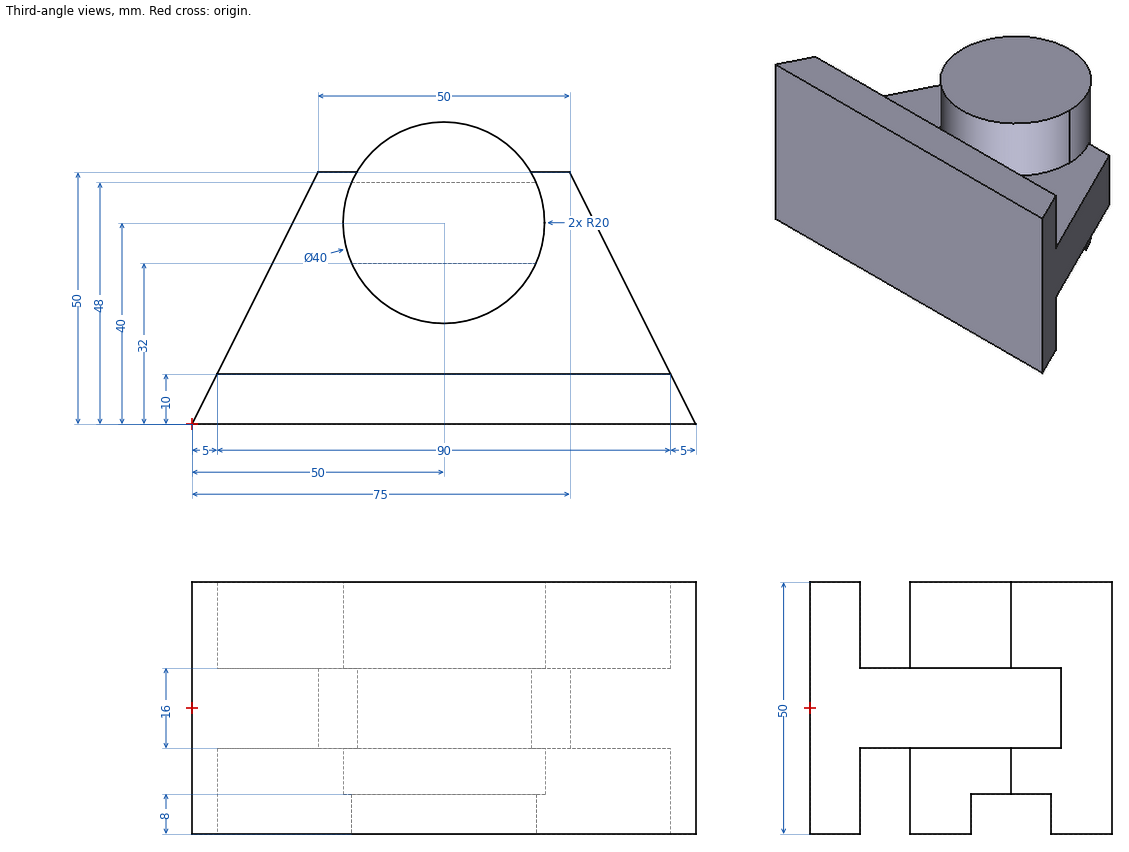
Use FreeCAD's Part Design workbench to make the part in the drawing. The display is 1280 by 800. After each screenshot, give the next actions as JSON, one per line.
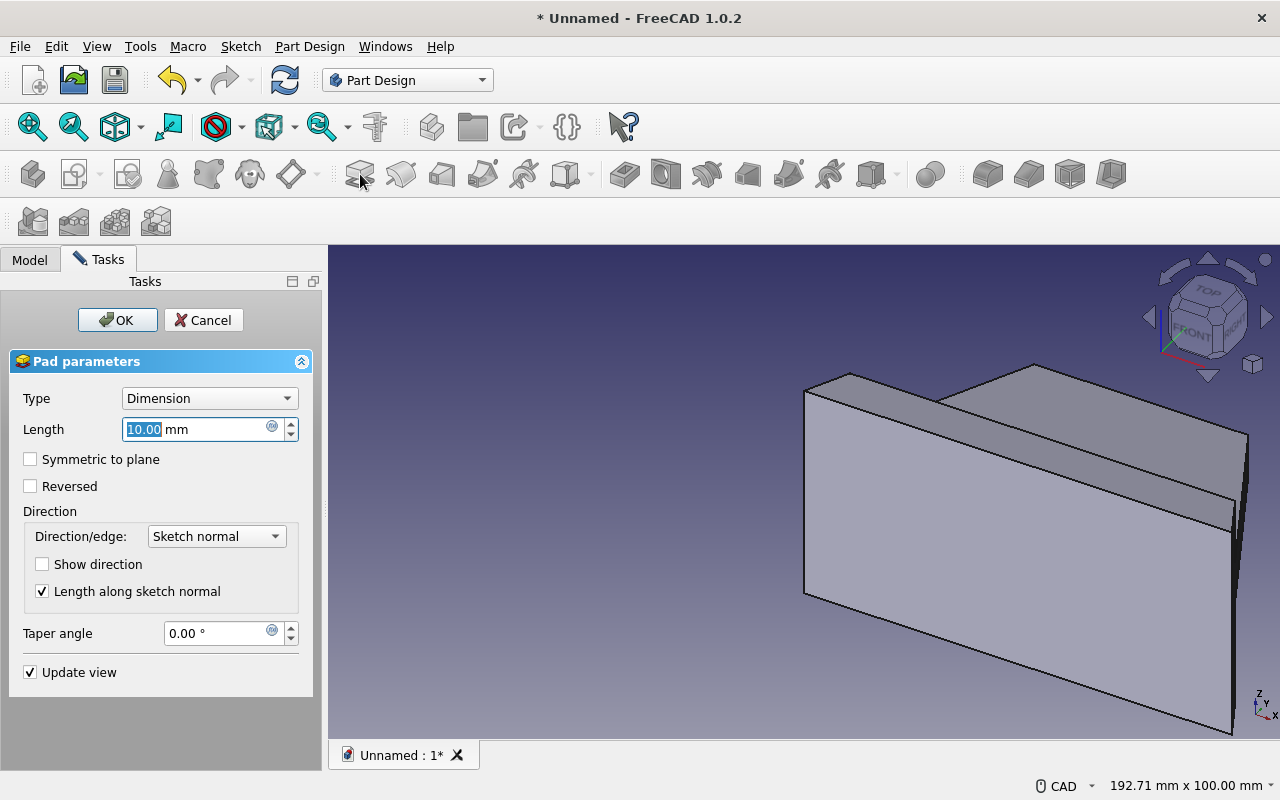
{"action": "type", "text": "16"}
{"action": "key", "text": "Tab"}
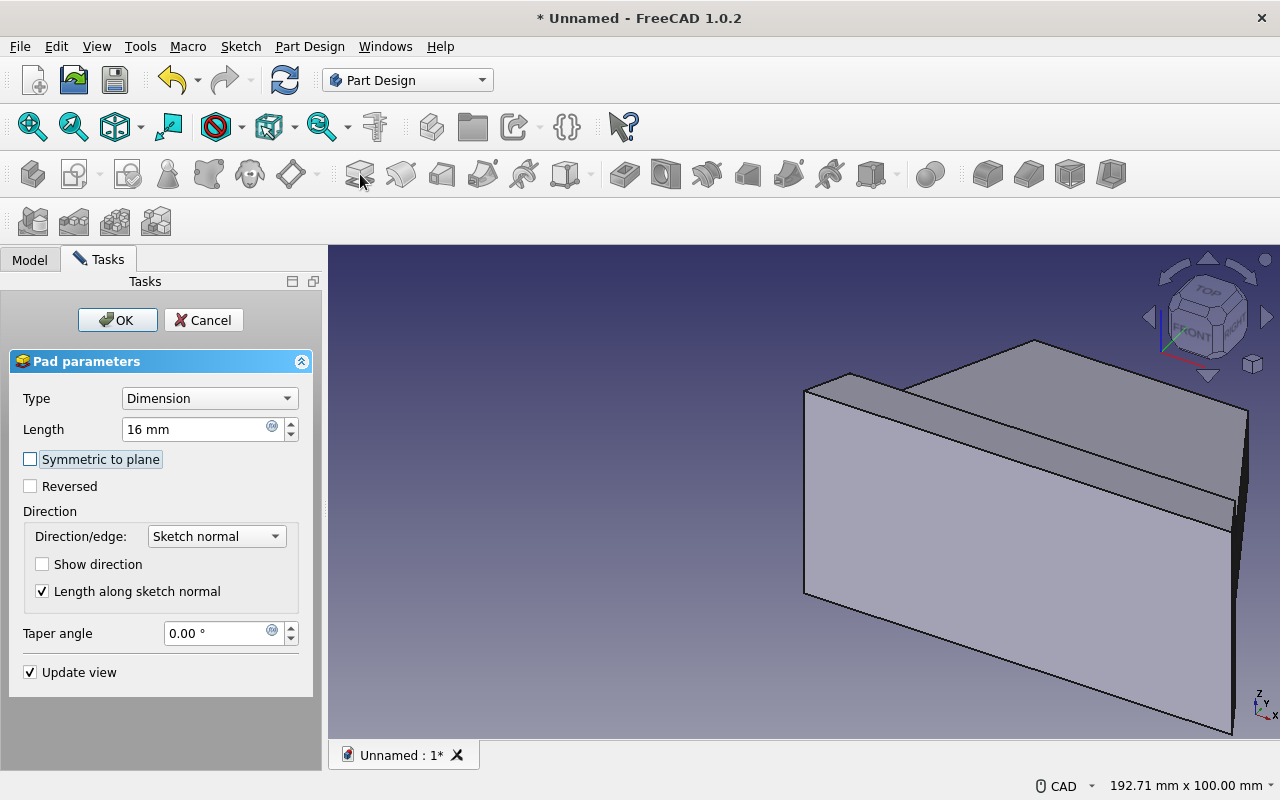
{"action": "left_click", "coordinate": [31, 459]}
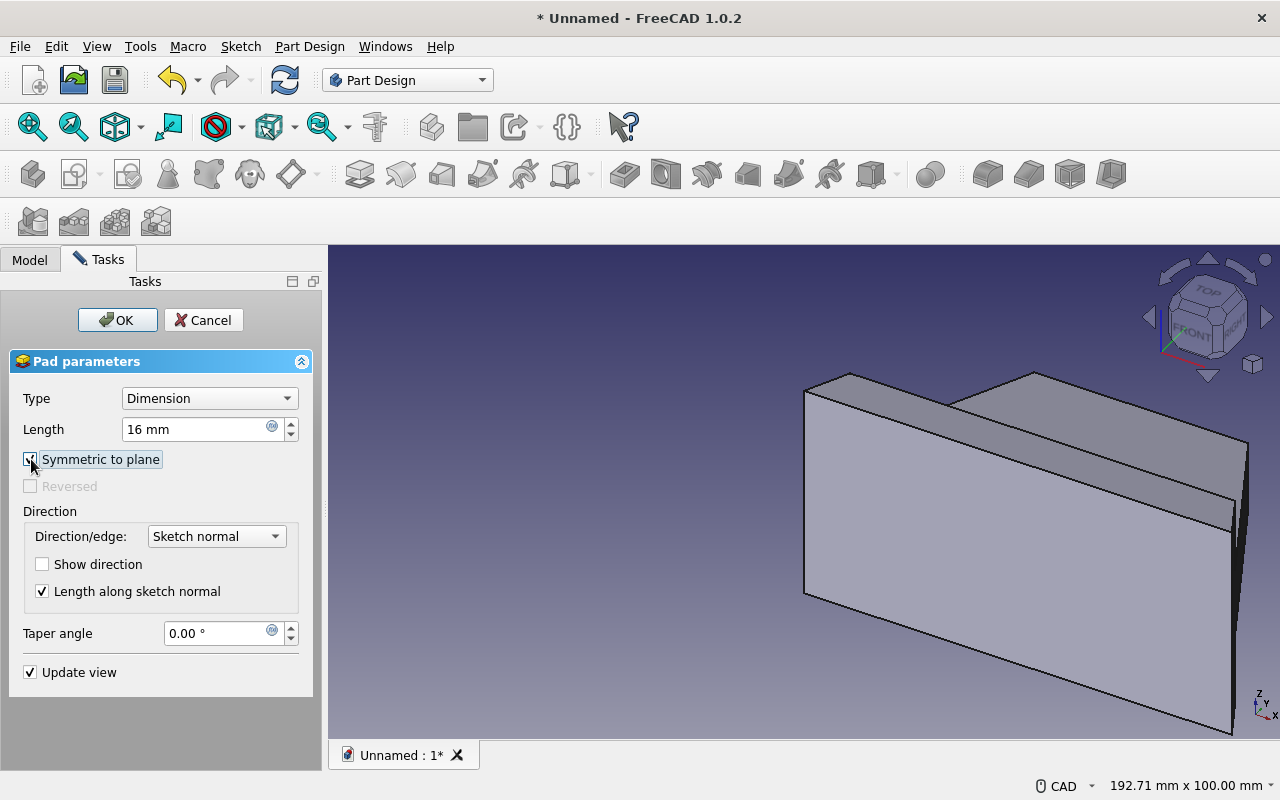
{"action": "left_click", "coordinate": [118, 320]}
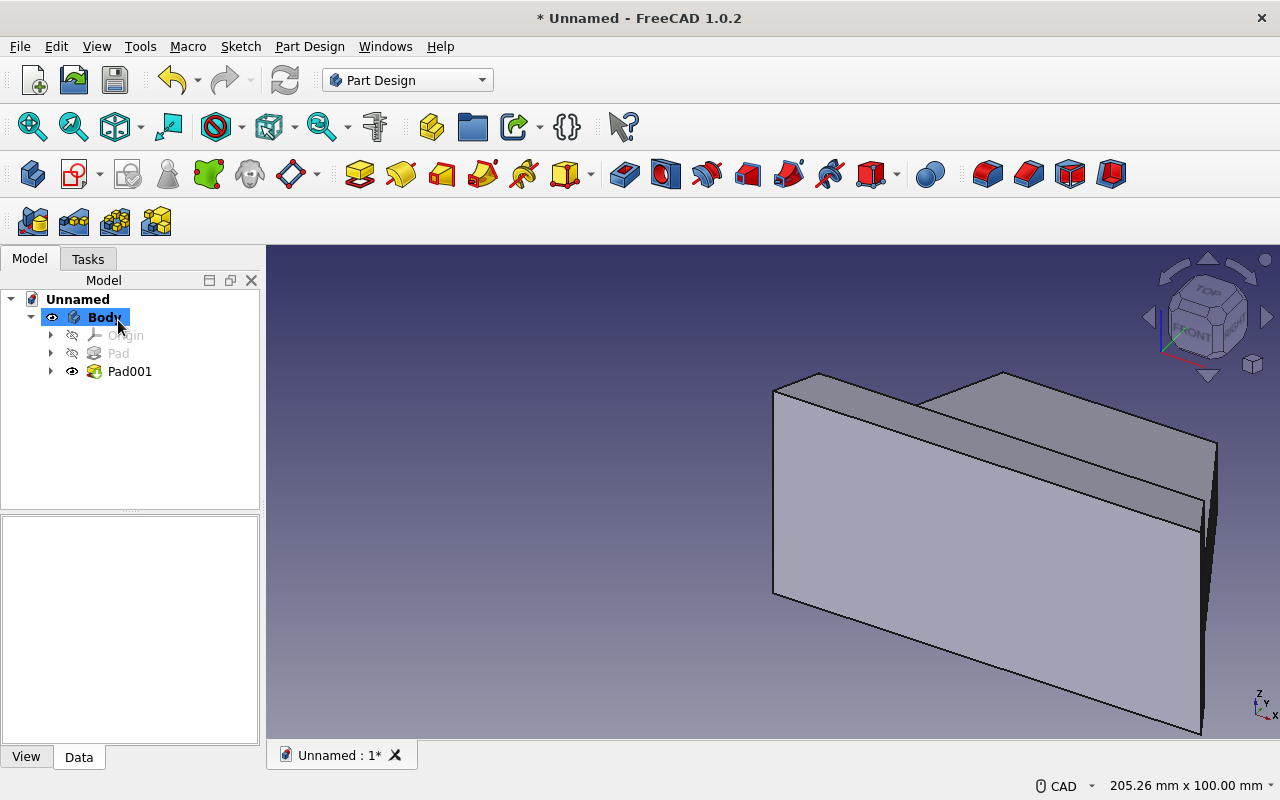
{"action": "left_click", "coordinate": [33, 128]}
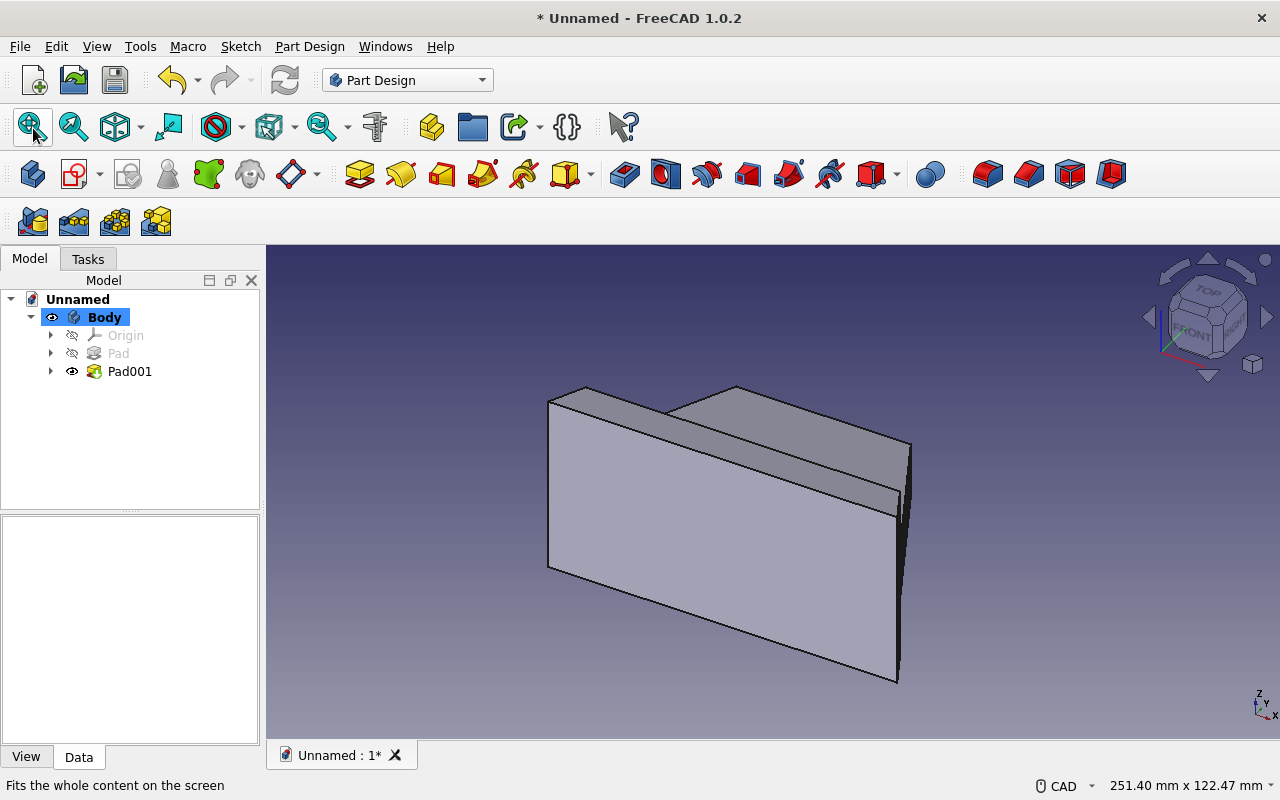
{"action": "left_click", "coordinate": [74, 174]}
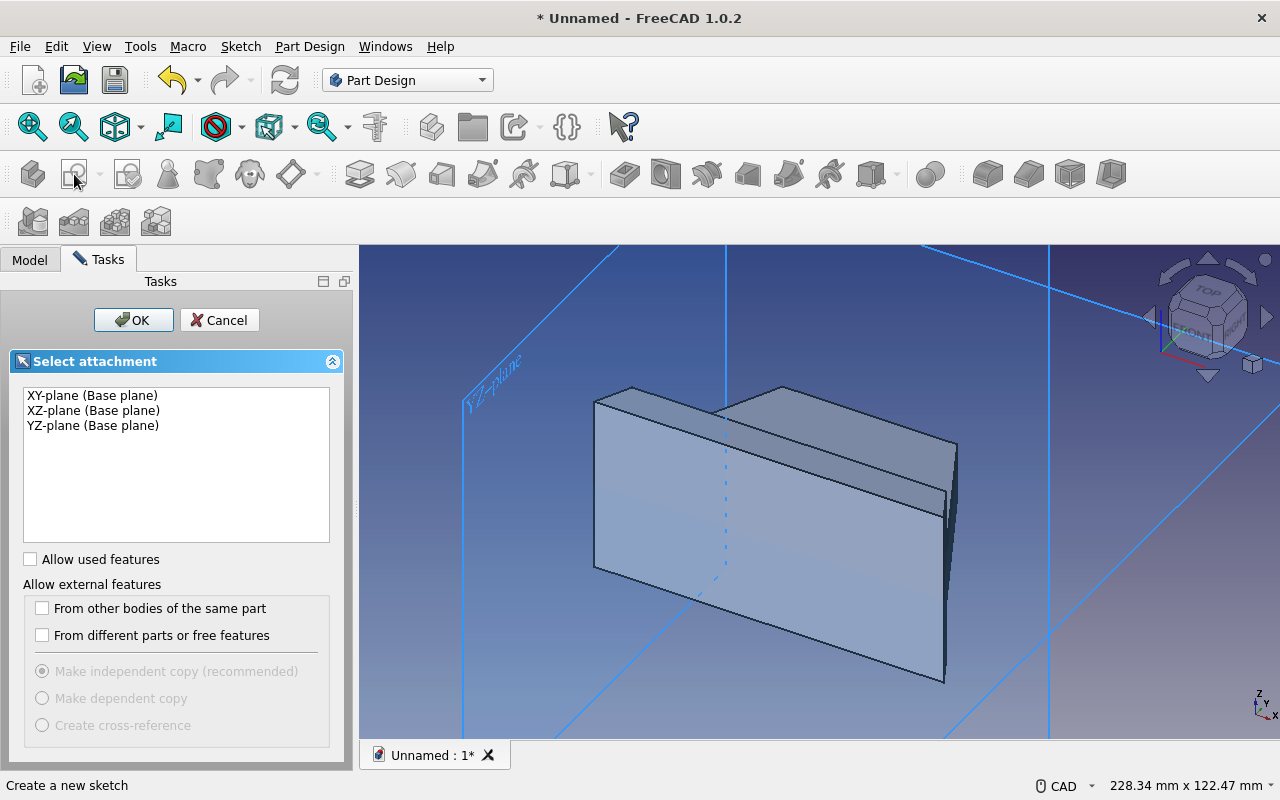
{"action": "left_click", "coordinate": [84, 396]}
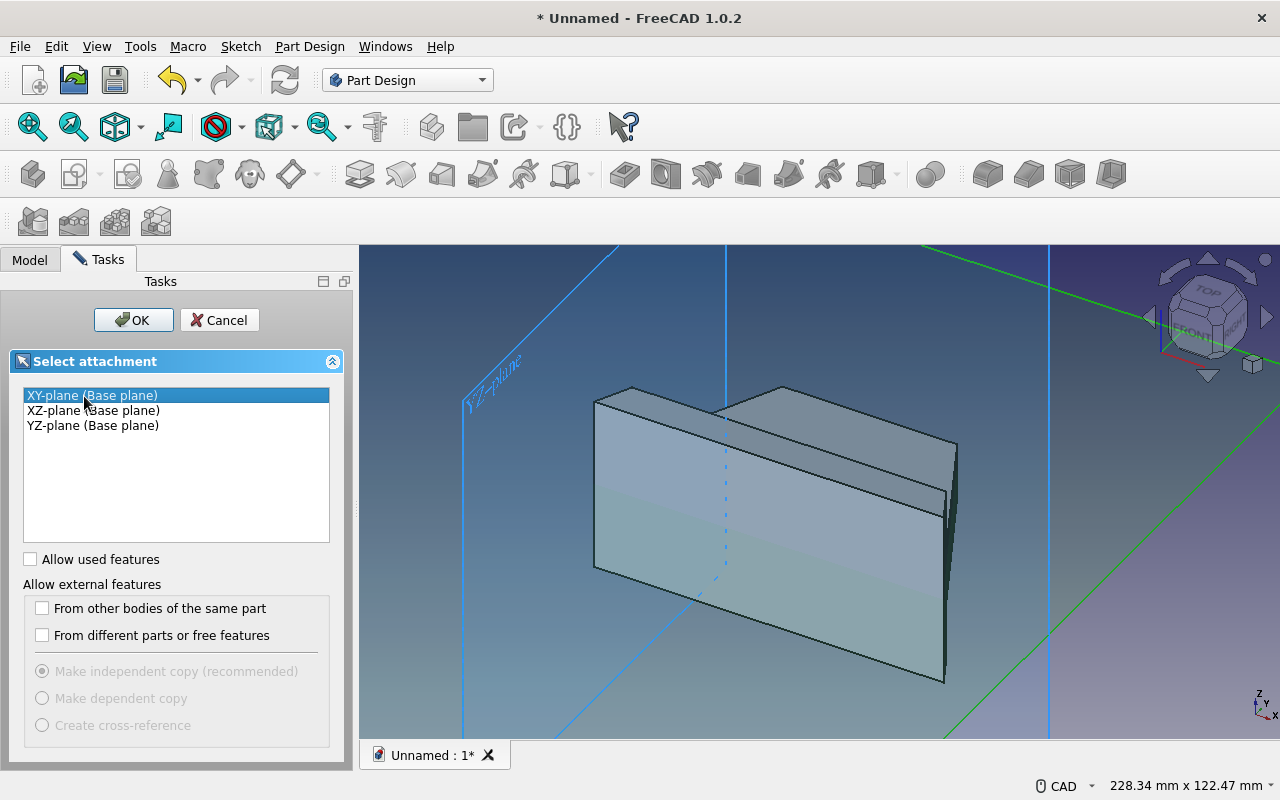
{"action": "left_click", "coordinate": [134, 320]}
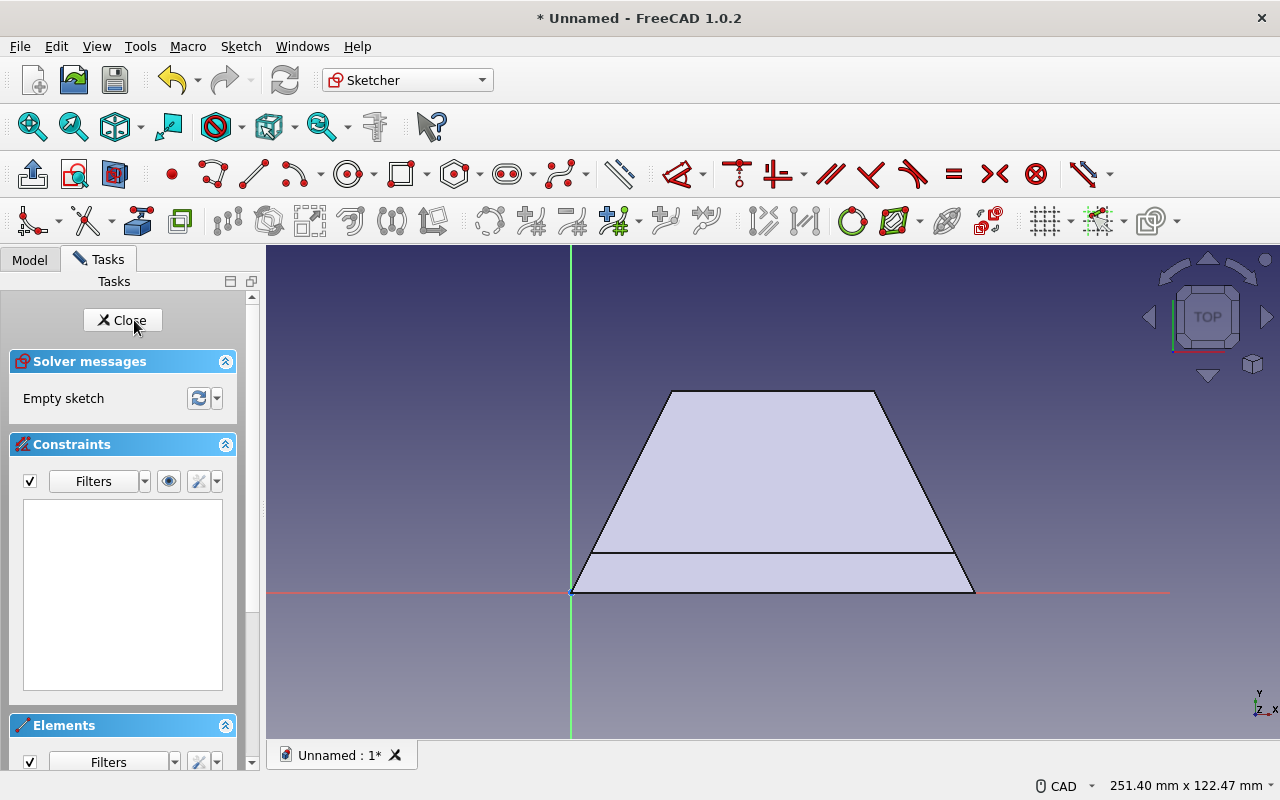
{"action": "left_click", "coordinate": [115, 174]}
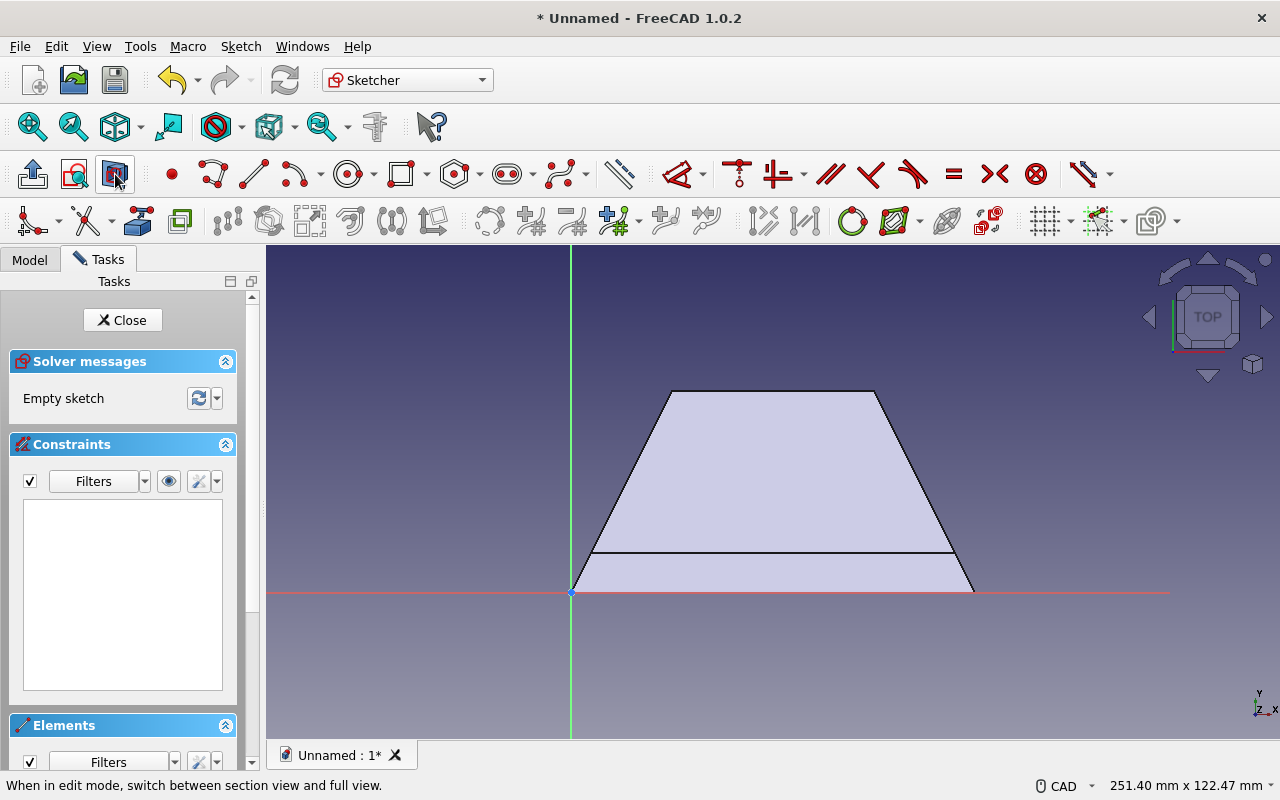
{"action": "left_click", "coordinate": [348, 174]}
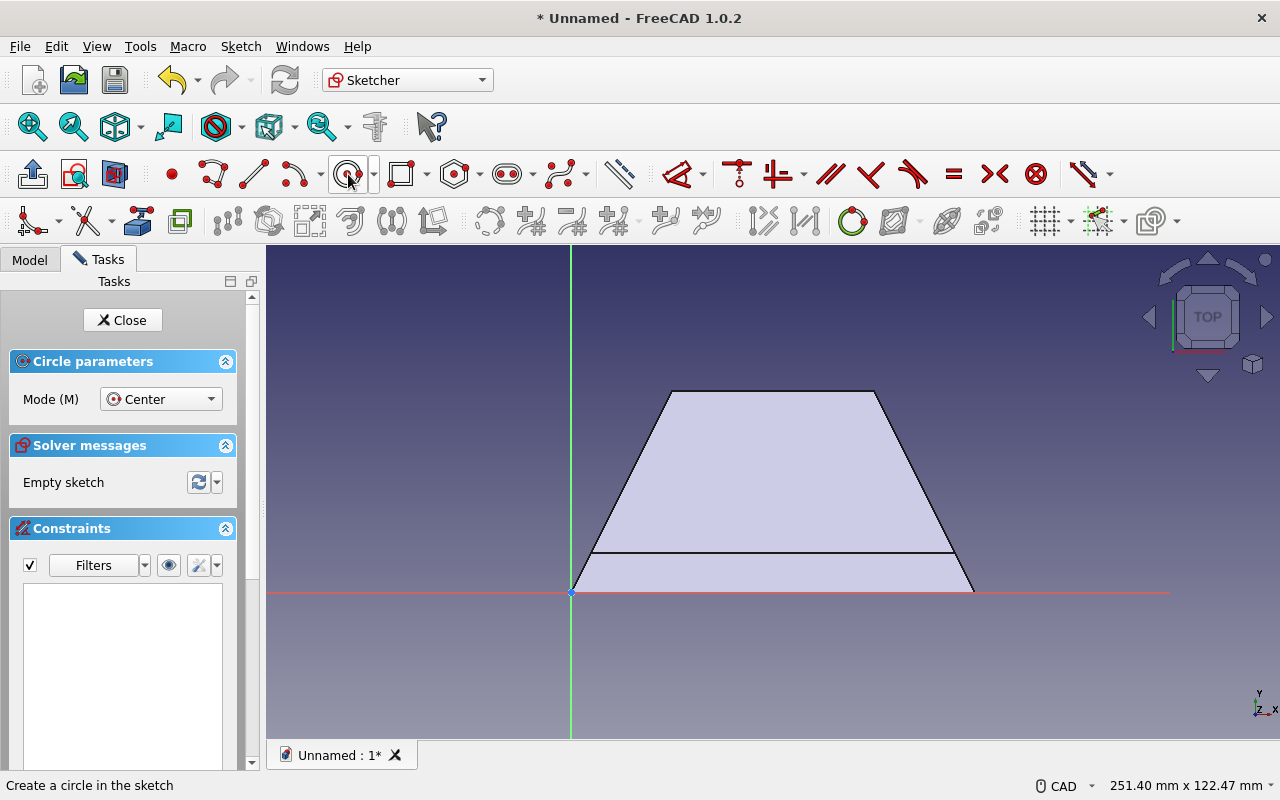
{"action": "left_click", "coordinate": [773, 431]}
{"action": "left_click", "coordinate": [830, 374]}
{"action": "key", "text": "Escape"}